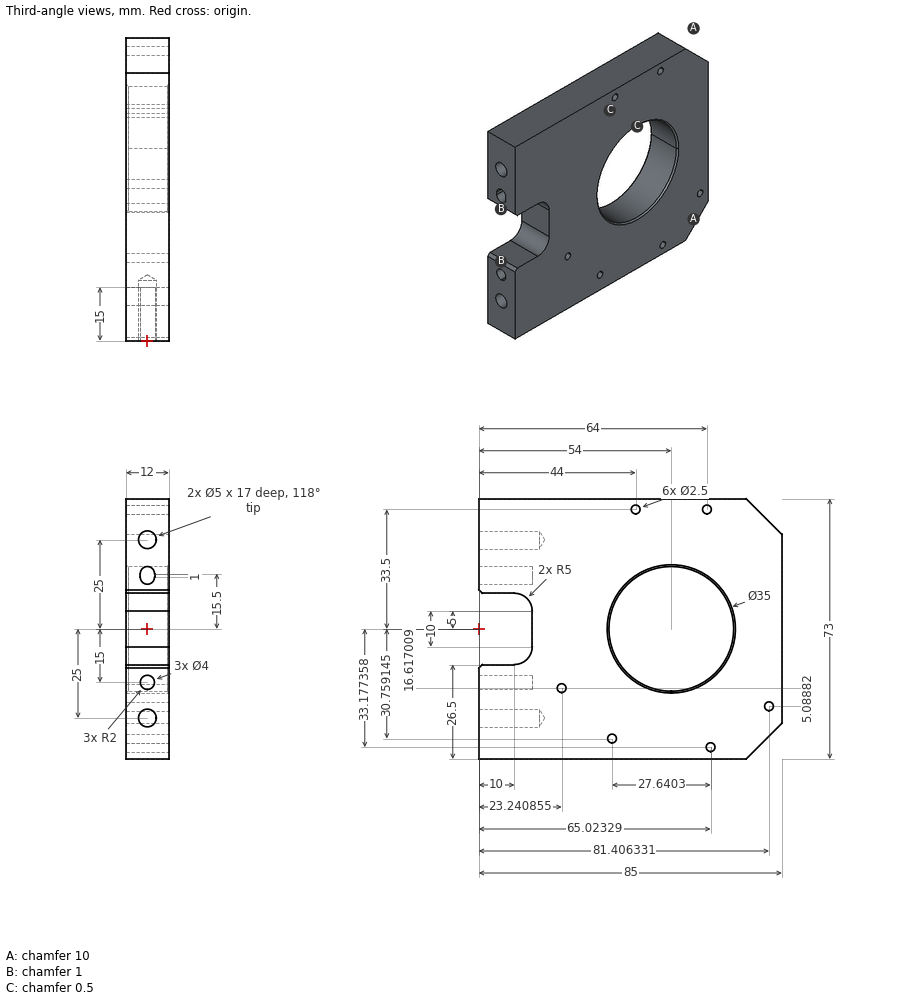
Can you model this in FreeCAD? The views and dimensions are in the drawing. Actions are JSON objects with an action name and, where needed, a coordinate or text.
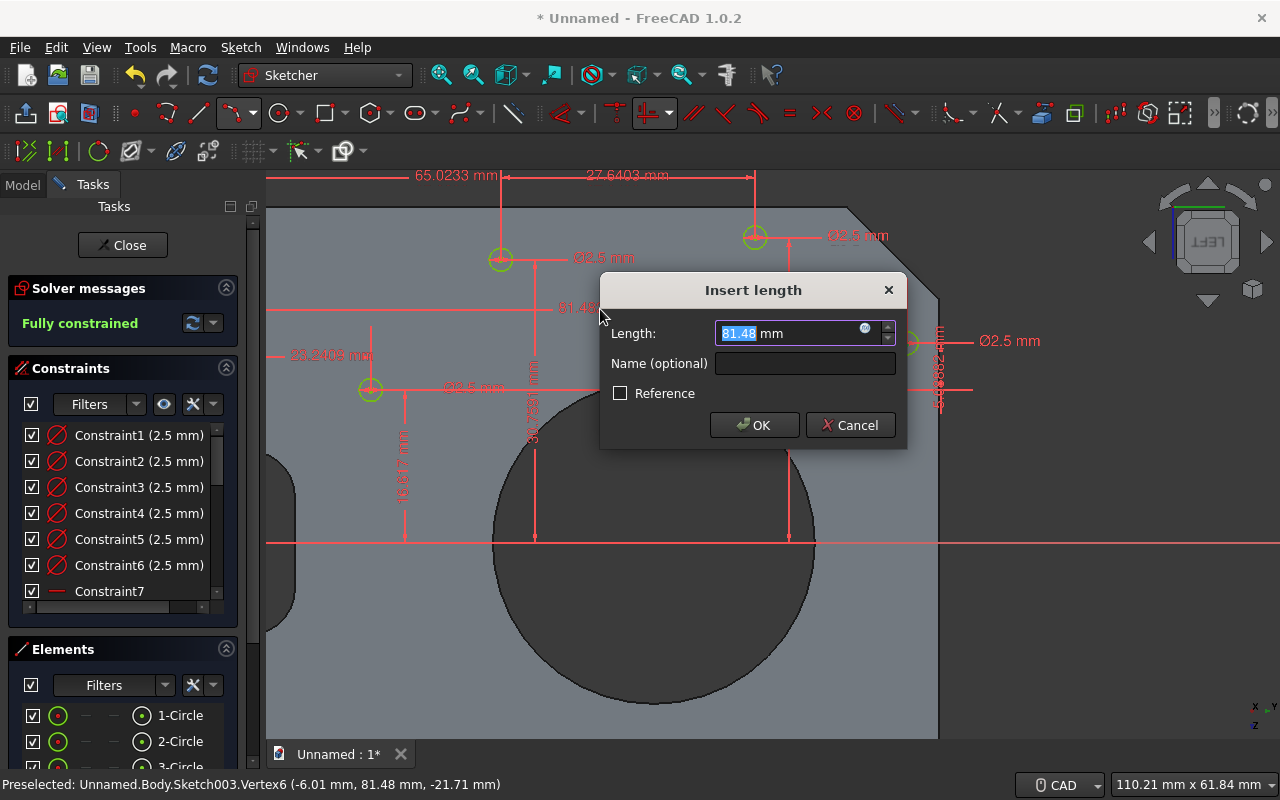
{"action": "type", "text": "81.406331"}
{"action": "key", "text": "Return"}
{"action": "key", "text": "Escape"}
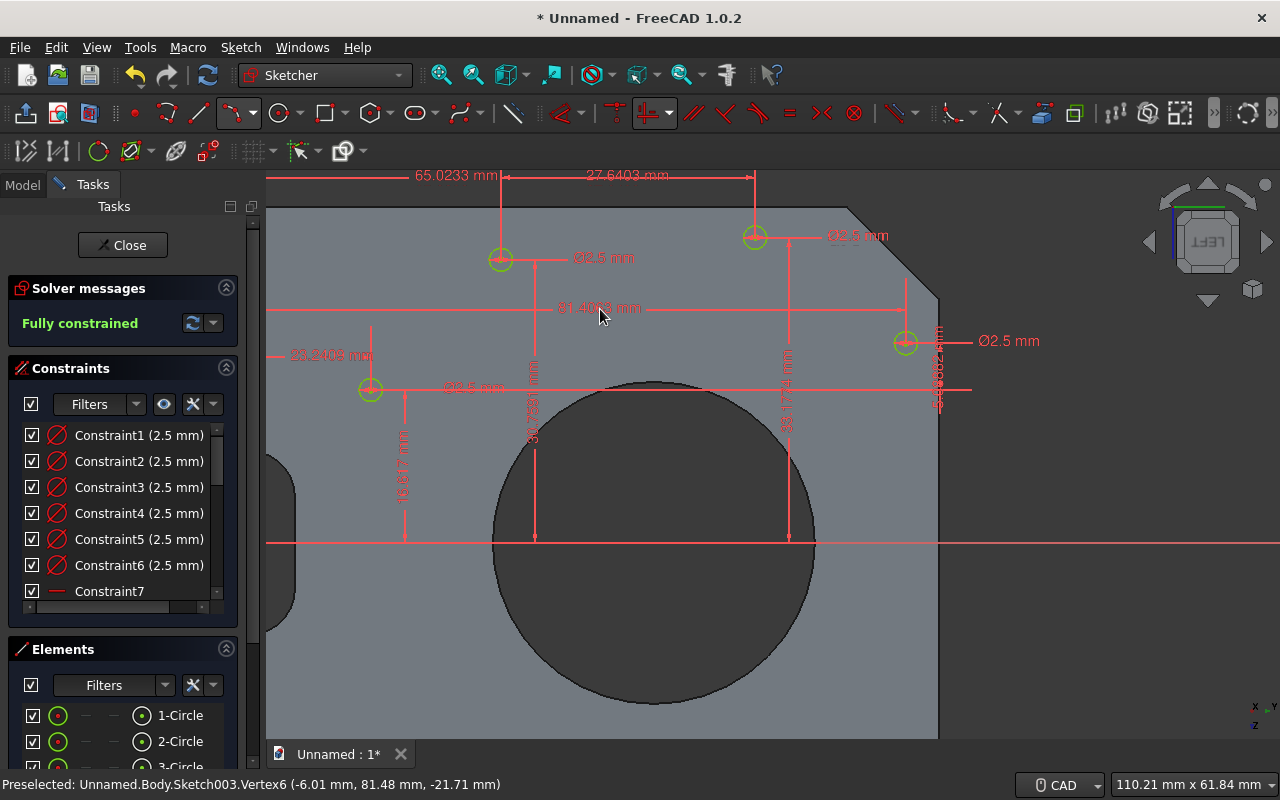
{"action": "left_click", "coordinate": [123, 245]}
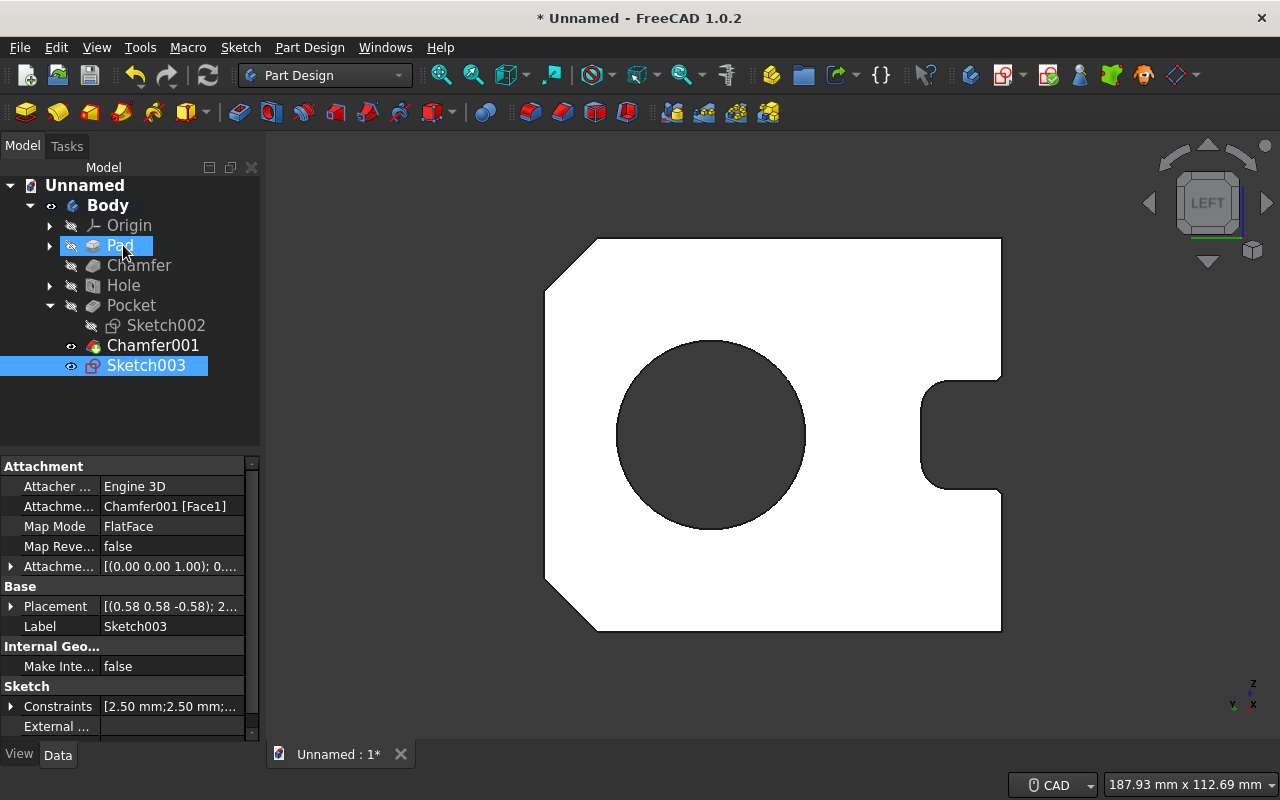
{"action": "left_click", "coordinate": [240, 112]}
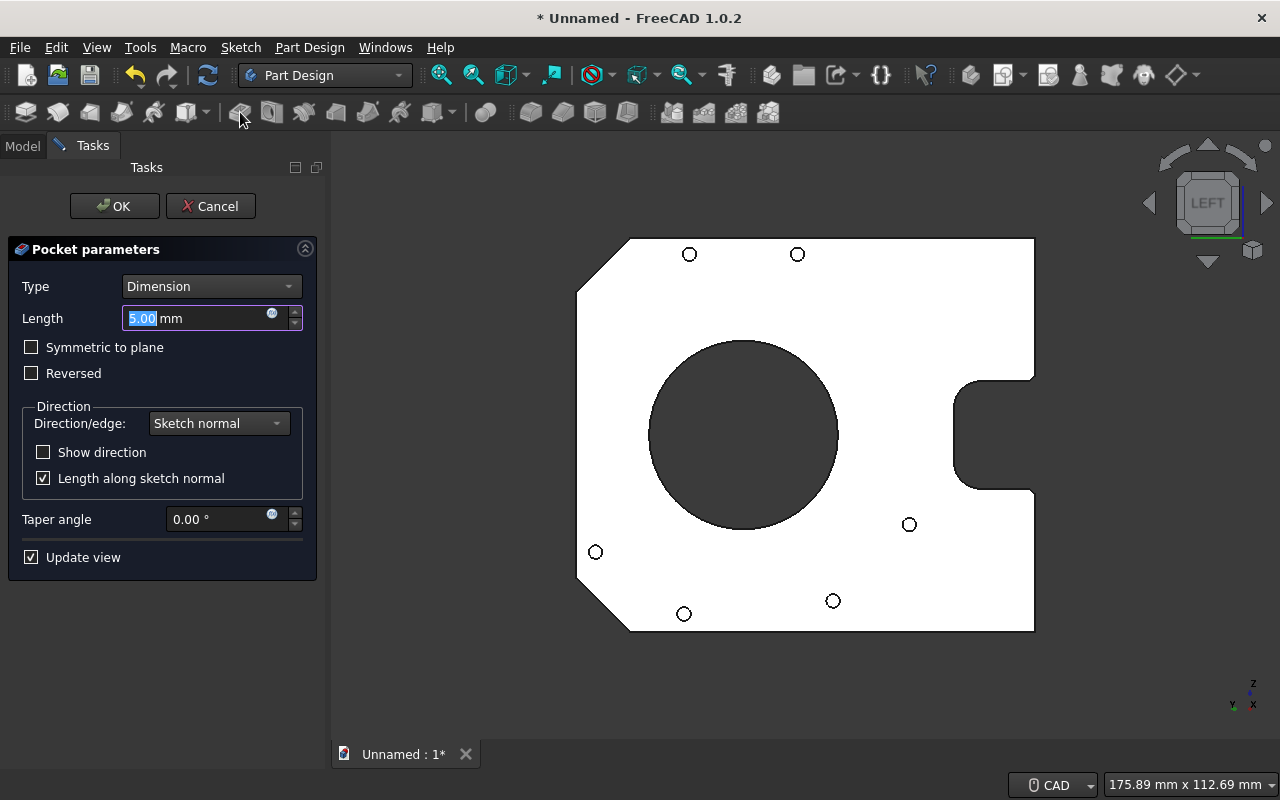
{"action": "left_click", "coordinate": [212, 286]}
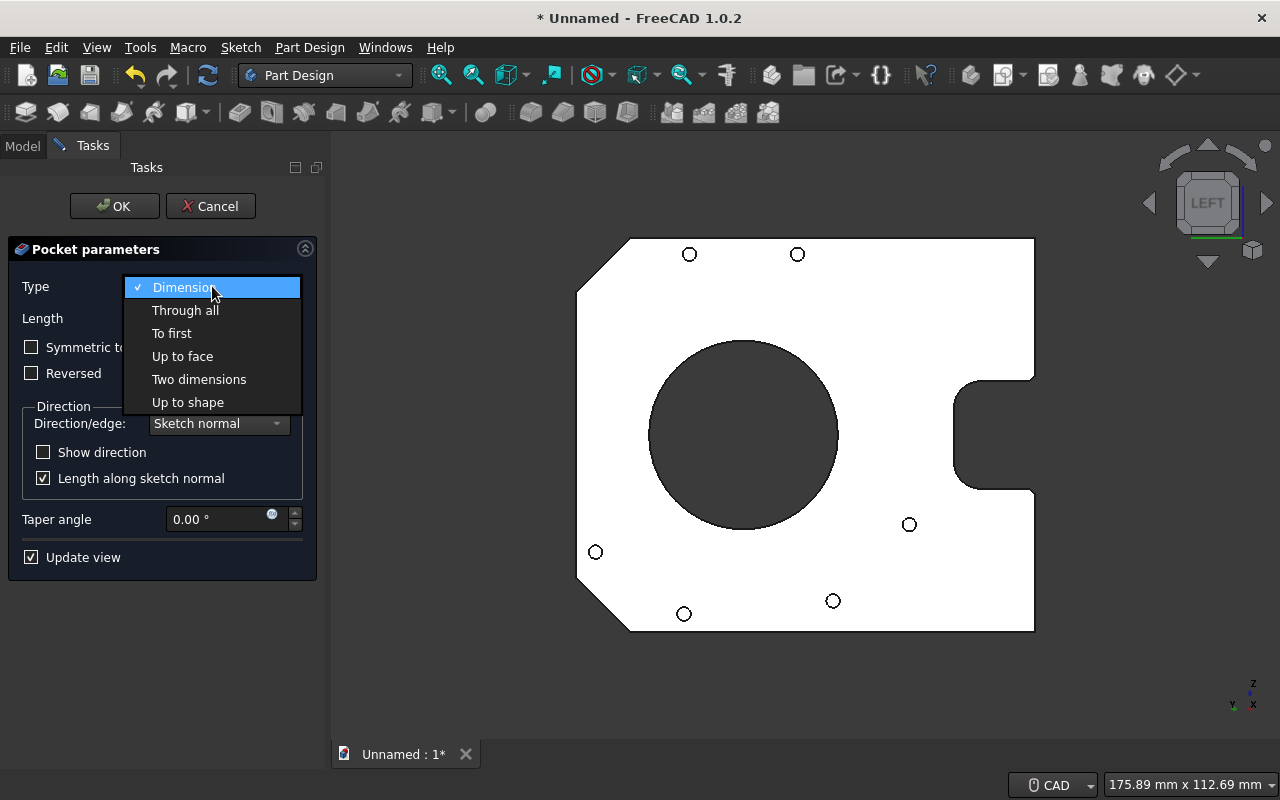
{"action": "left_click", "coordinate": [212, 310]}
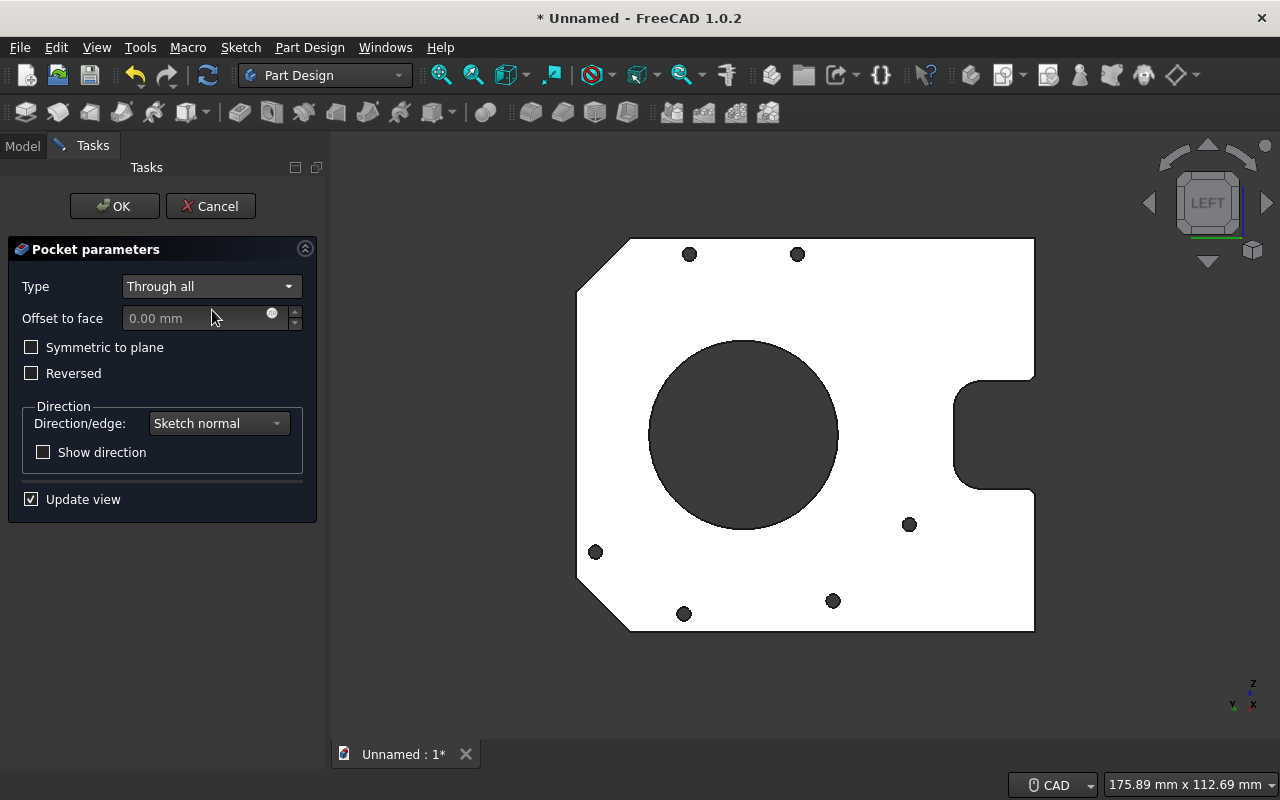
{"action": "left_click", "coordinate": [115, 206]}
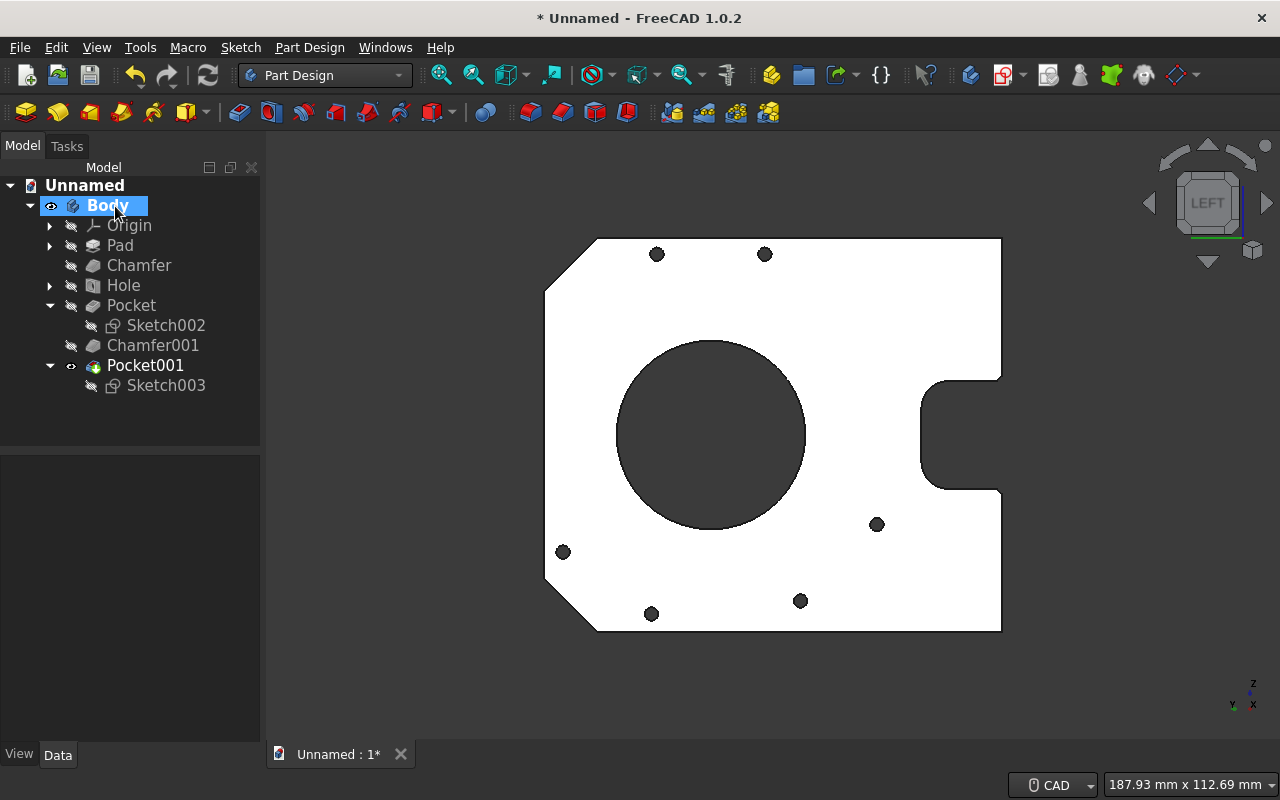
{"action": "left_click", "coordinate": [805, 434]}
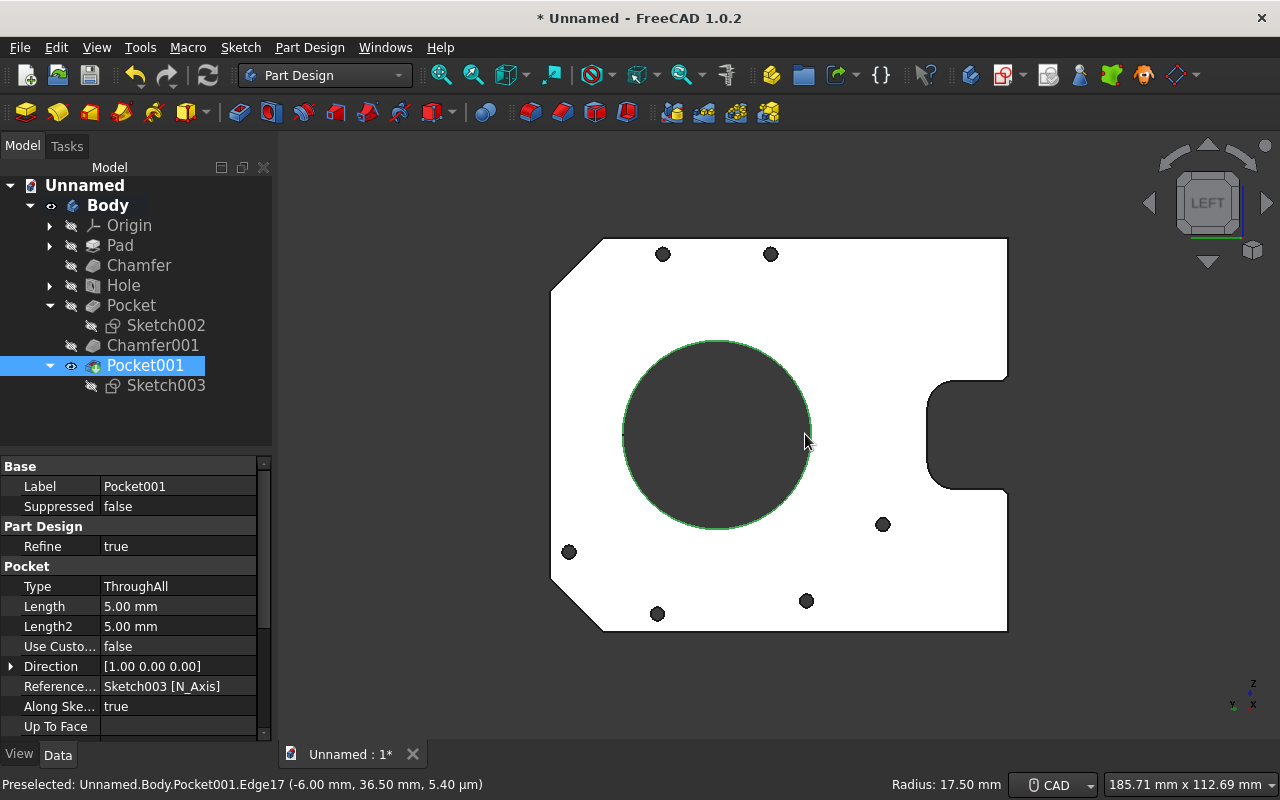
{"action": "key", "text": "0"}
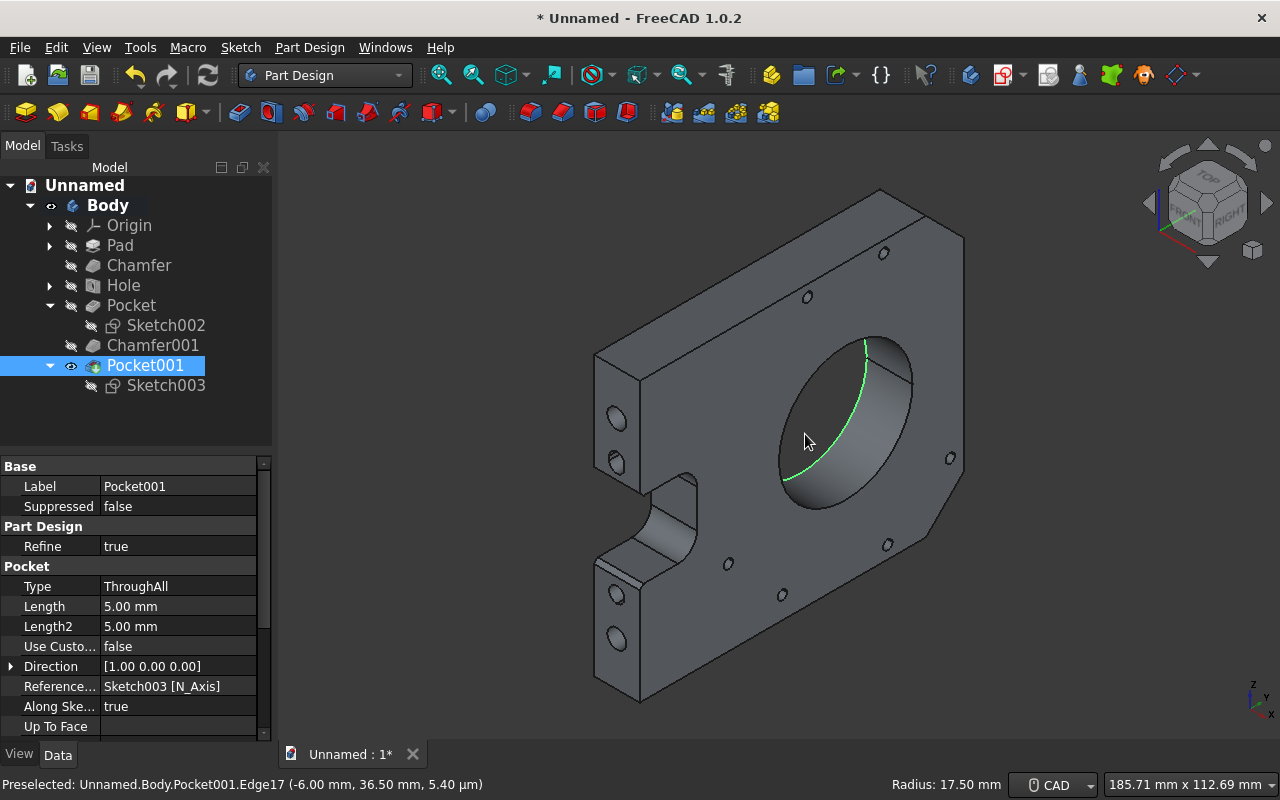
{"action": "left_click", "coordinate": [825, 507], "text": "ctrl"}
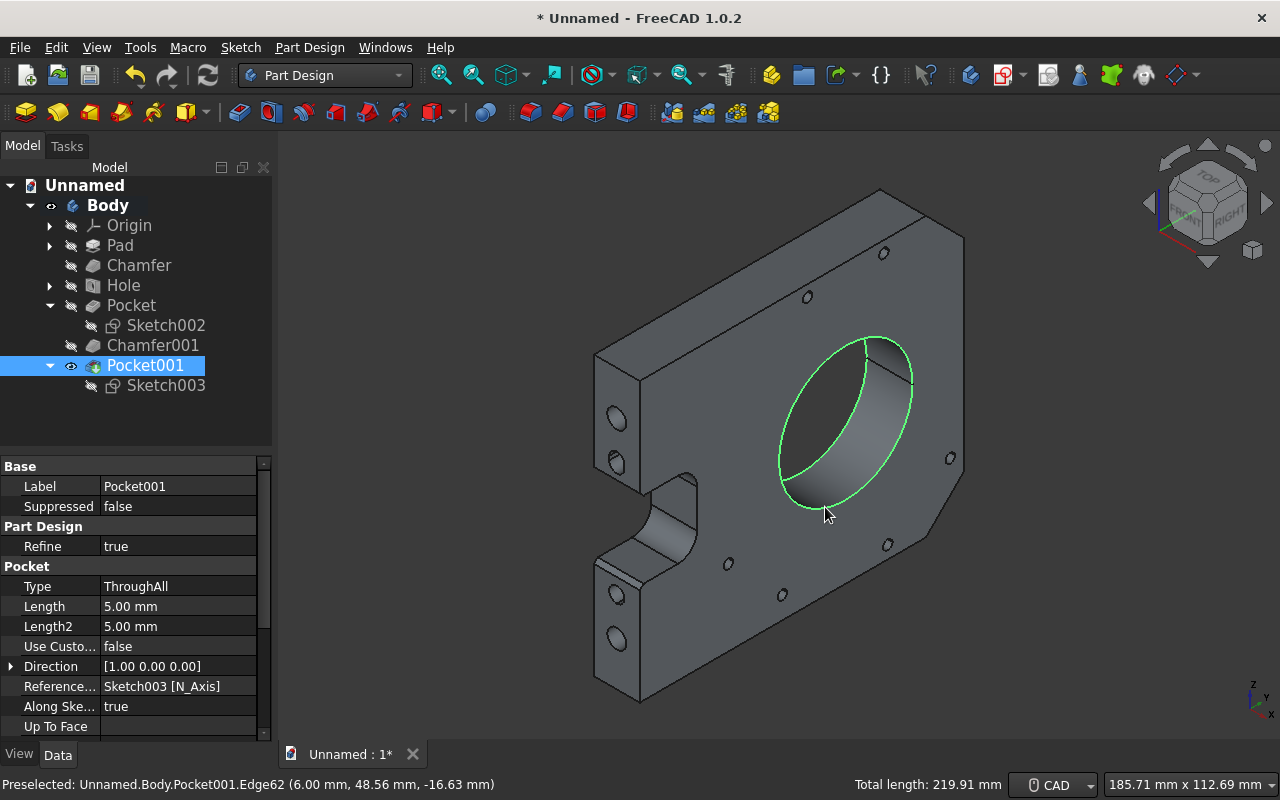
{"action": "left_click", "coordinate": [564, 112]}